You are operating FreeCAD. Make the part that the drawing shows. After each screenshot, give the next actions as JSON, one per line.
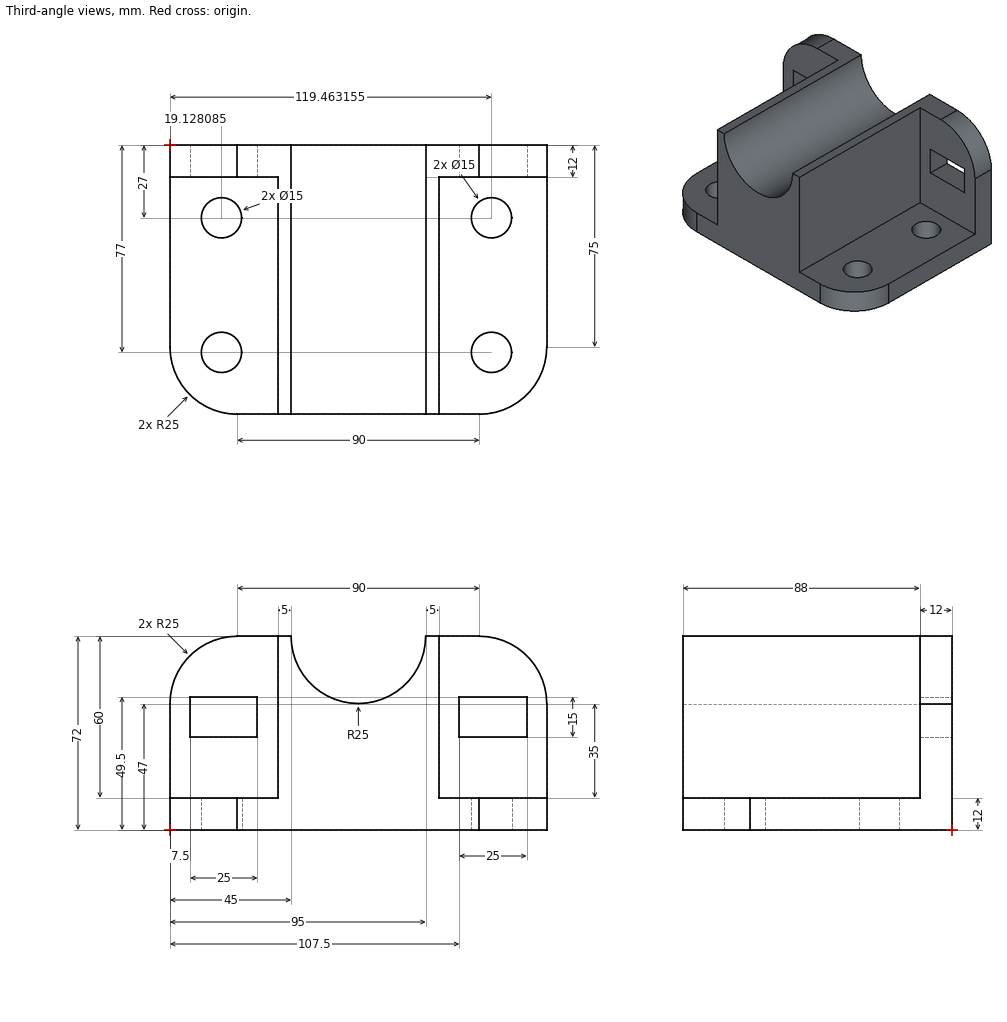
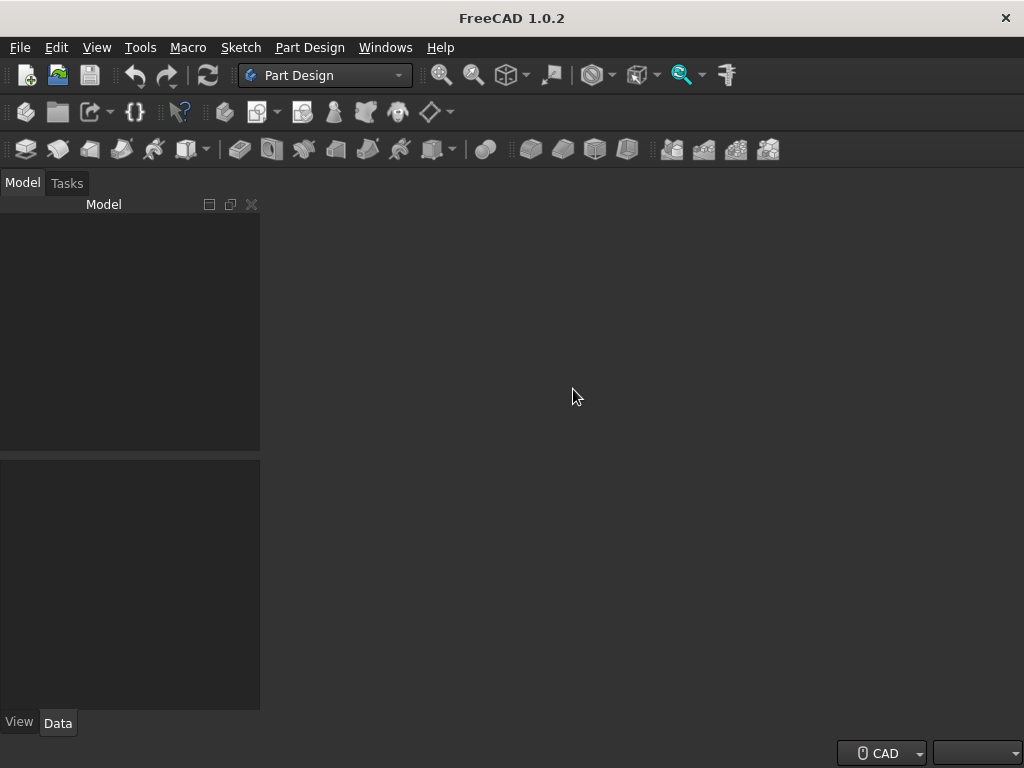
{"action": "left_click", "coordinate": [26, 76]}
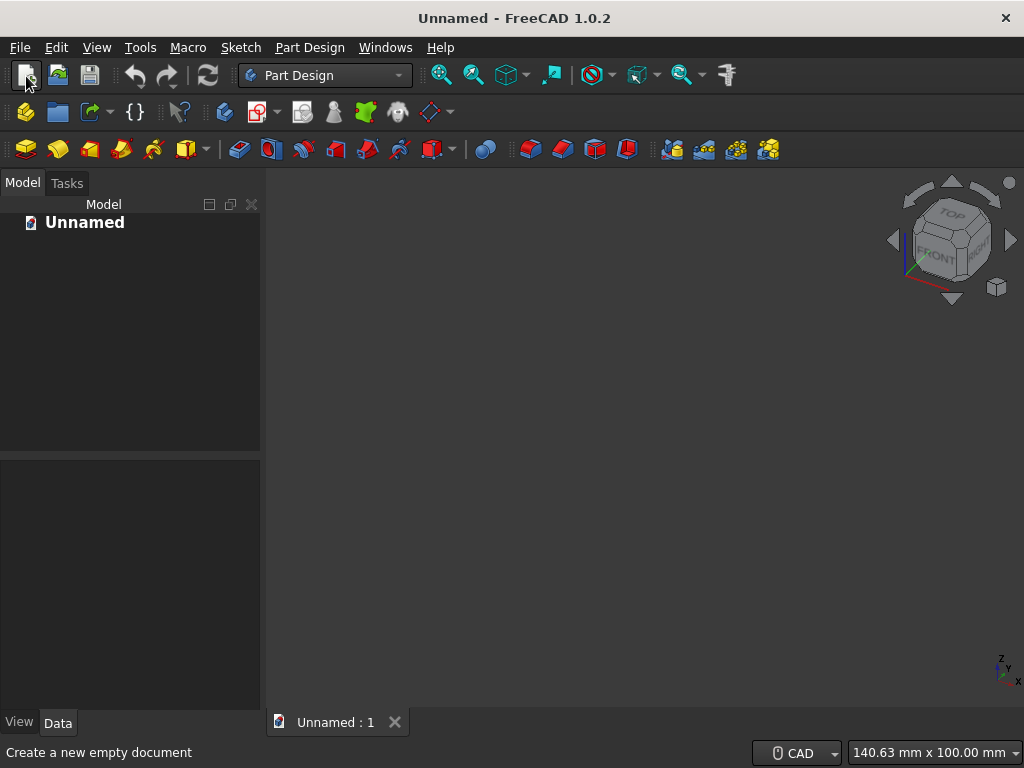
{"action": "left_click", "coordinate": [258, 112]}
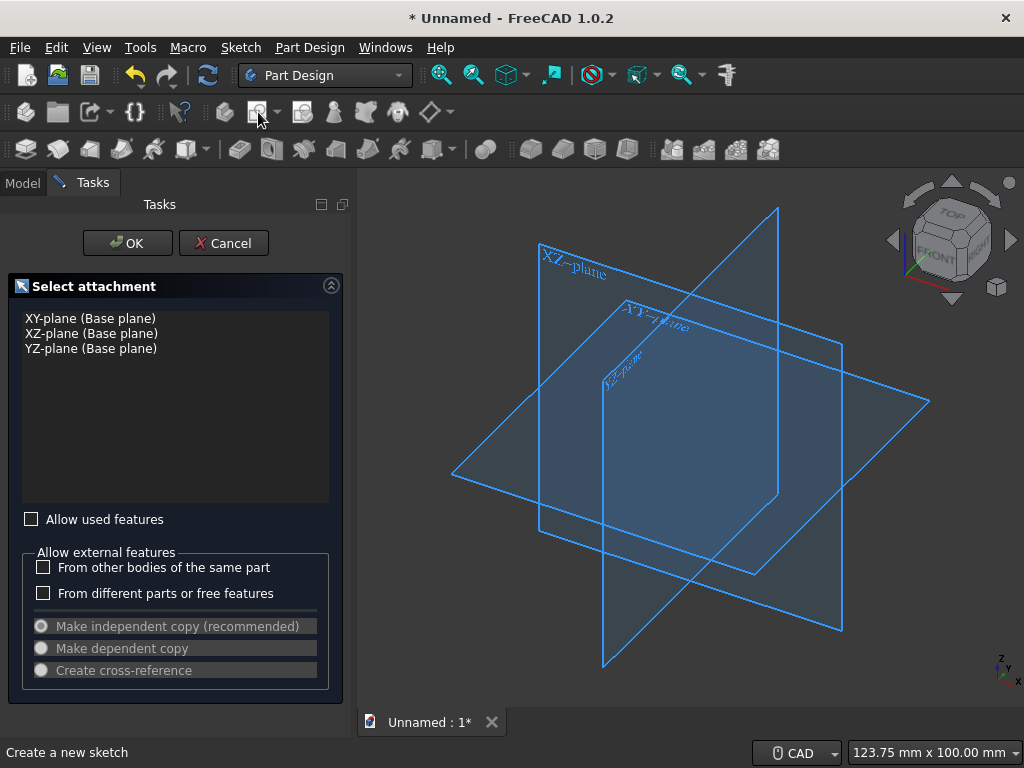
{"action": "left_click", "coordinate": [82, 318]}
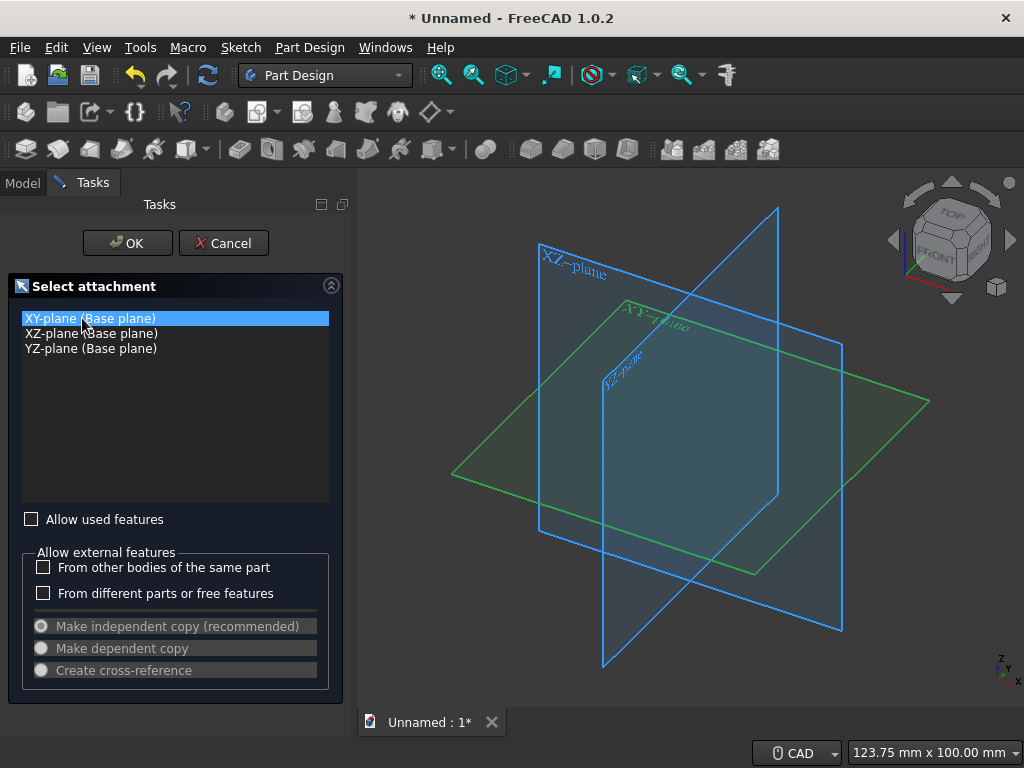
{"action": "left_click", "coordinate": [128, 243]}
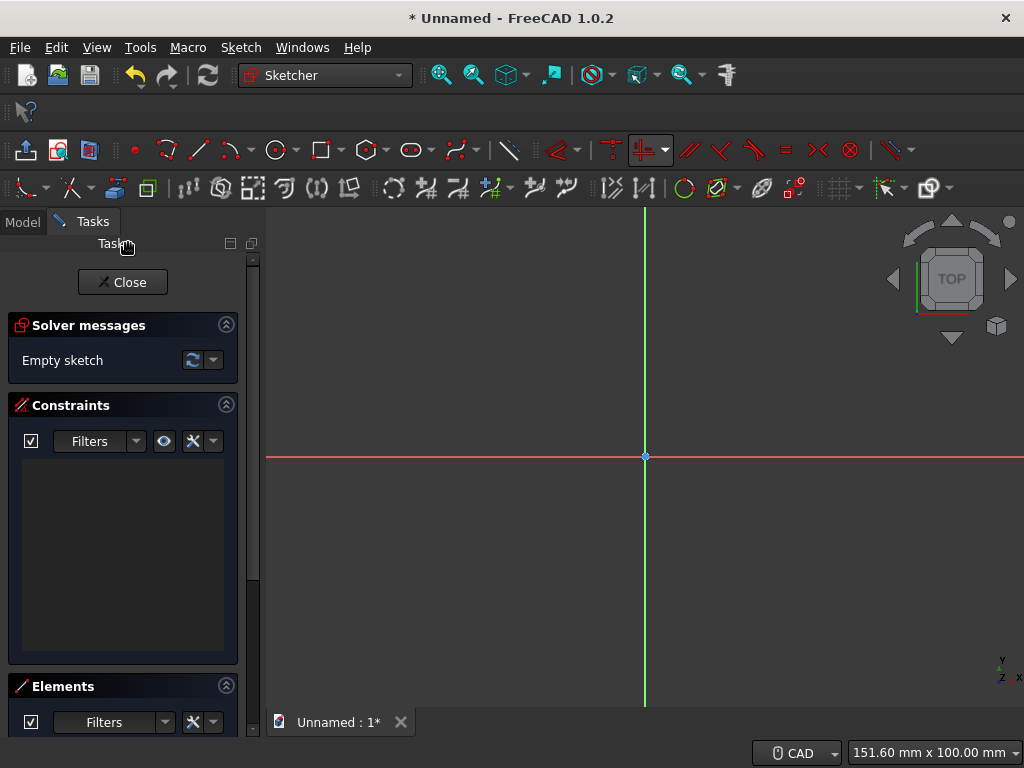
{"action": "scroll", "coordinate": [294, 253], "scroll_direction": "down", "scroll_amount": 4}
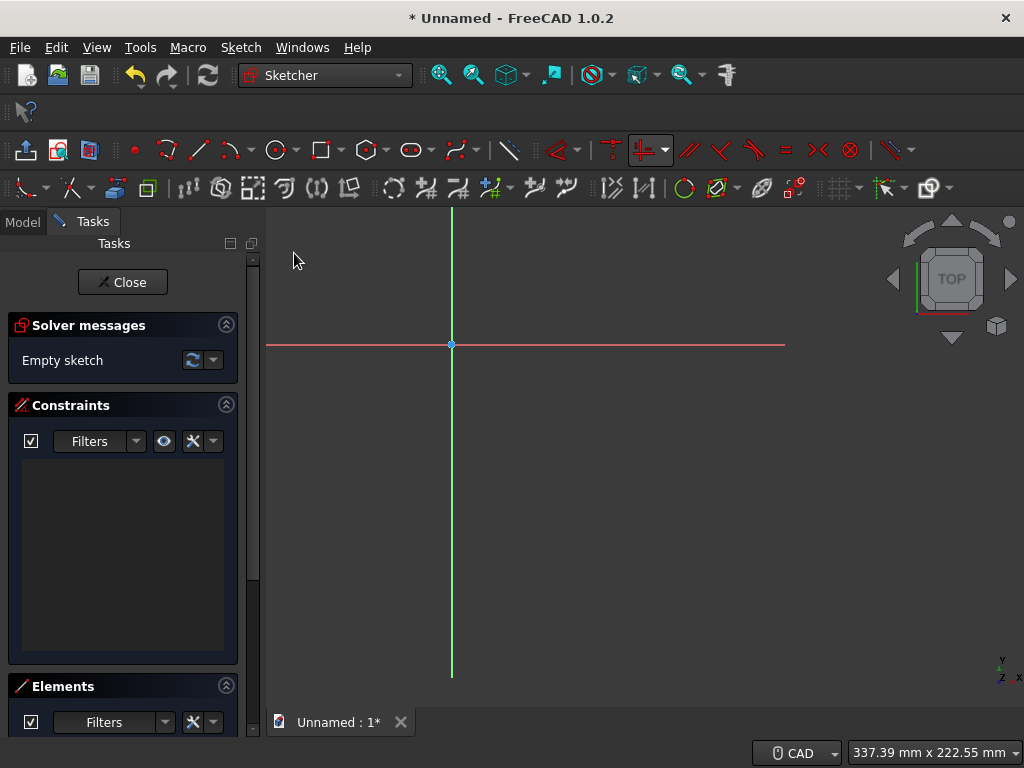
{"action": "left_click", "coordinate": [200, 150]}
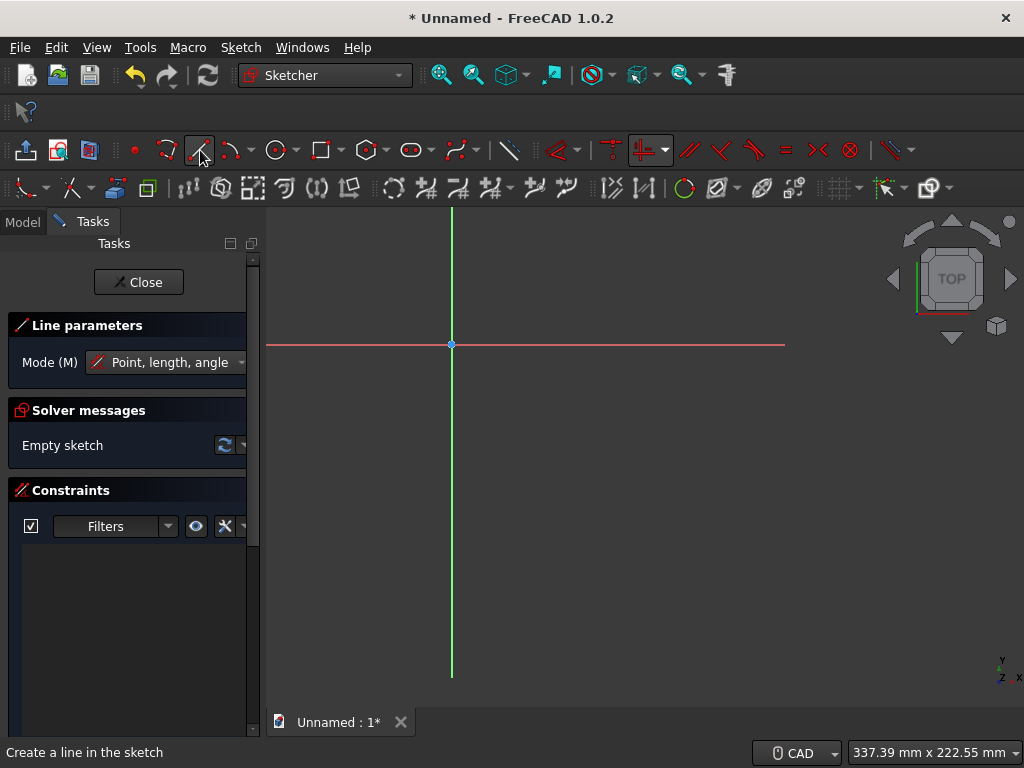
{"action": "left_click", "coordinate": [508, 569]}
{"action": "left_click", "coordinate": [710, 569]}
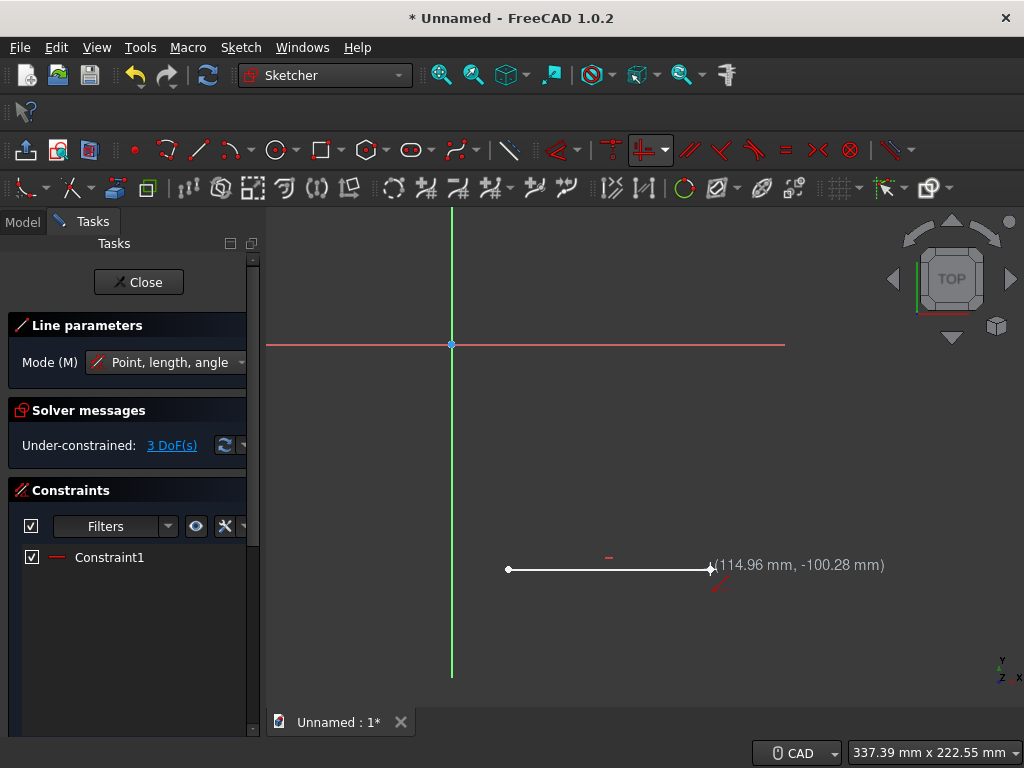
{"action": "left_click", "coordinate": [168, 150]}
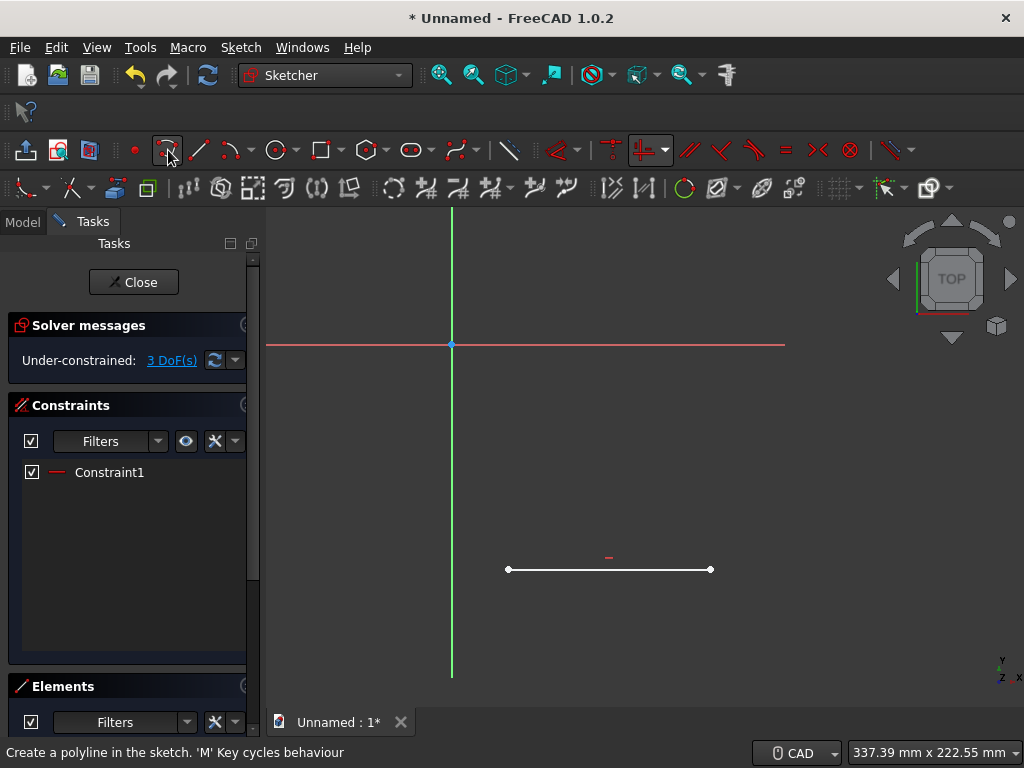
{"action": "left_click", "coordinate": [766, 513]}
{"action": "left_click", "coordinate": [766, 345]}
{"action": "left_click", "coordinate": [452, 345]}
{"action": "left_click", "coordinate": [461, 513]}
{"action": "right_click", "coordinate": [461, 513]}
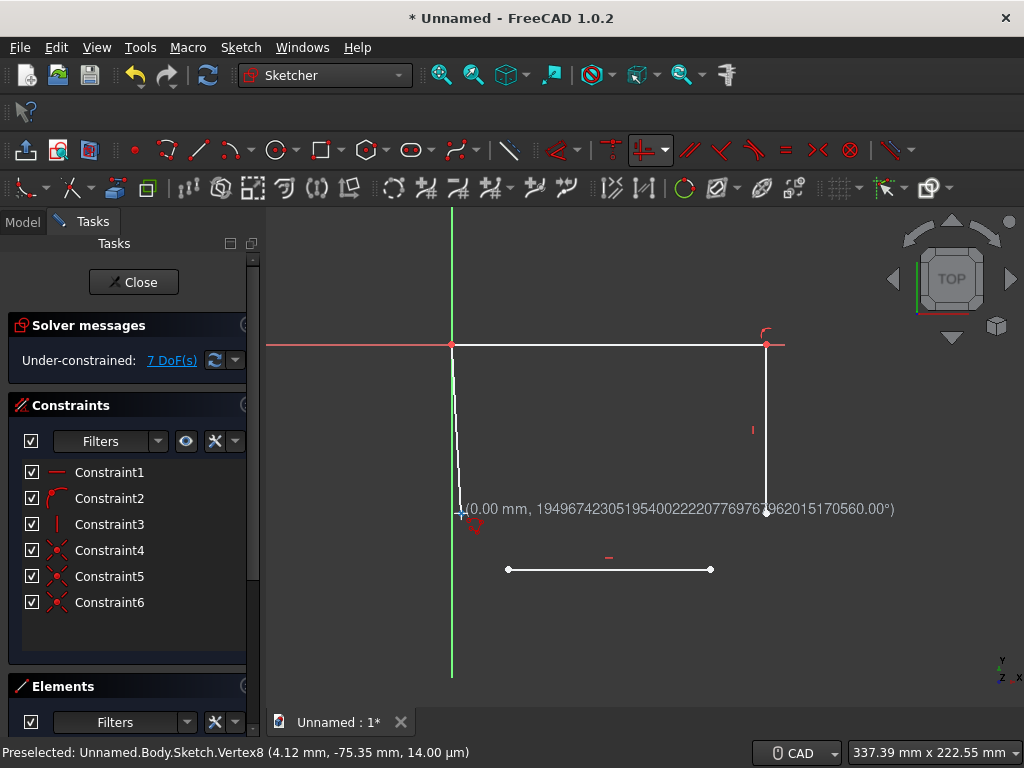
{"action": "key", "text": "g 3 a"}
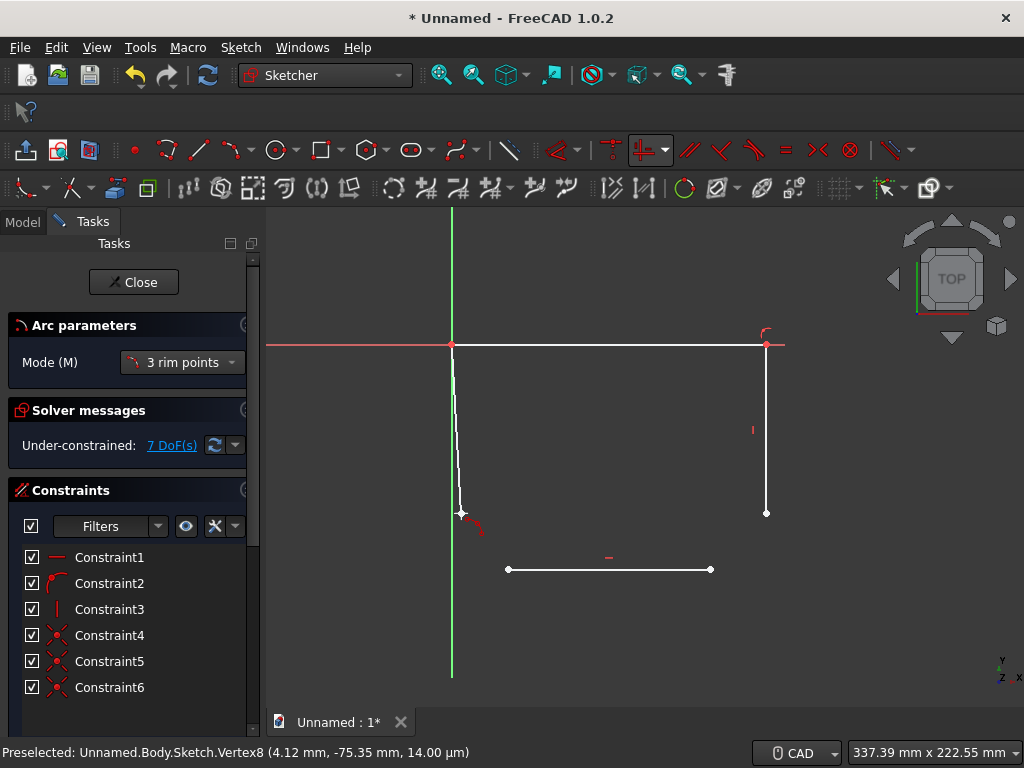
{"action": "left_click", "coordinate": [710, 570]}
{"action": "left_click", "coordinate": [766, 514]}
{"action": "left_click", "coordinate": [750, 553]}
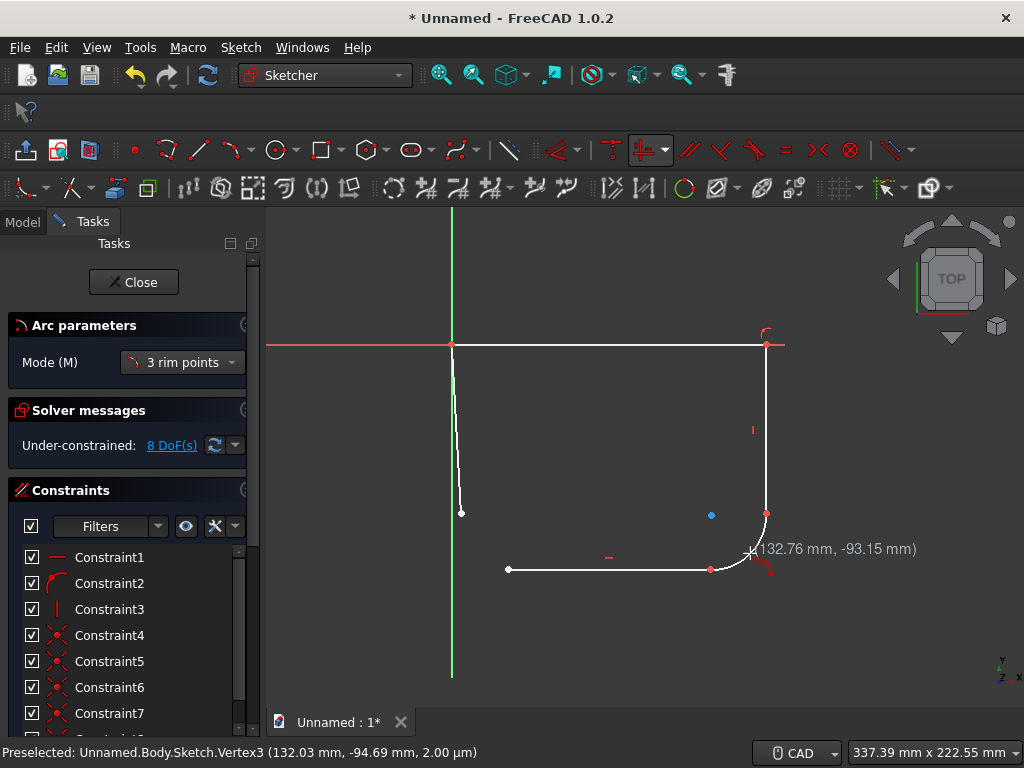
{"action": "left_click", "coordinate": [461, 514]}
{"action": "left_click", "coordinate": [508, 570]}
{"action": "left_click", "coordinate": [468, 553]}
{"action": "key", "text": "Escape"}